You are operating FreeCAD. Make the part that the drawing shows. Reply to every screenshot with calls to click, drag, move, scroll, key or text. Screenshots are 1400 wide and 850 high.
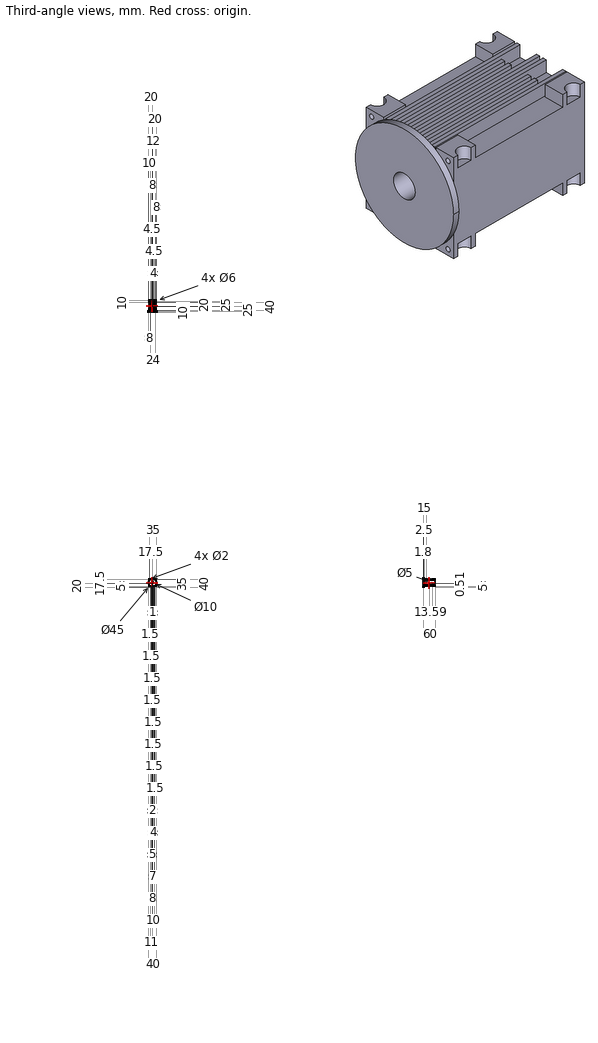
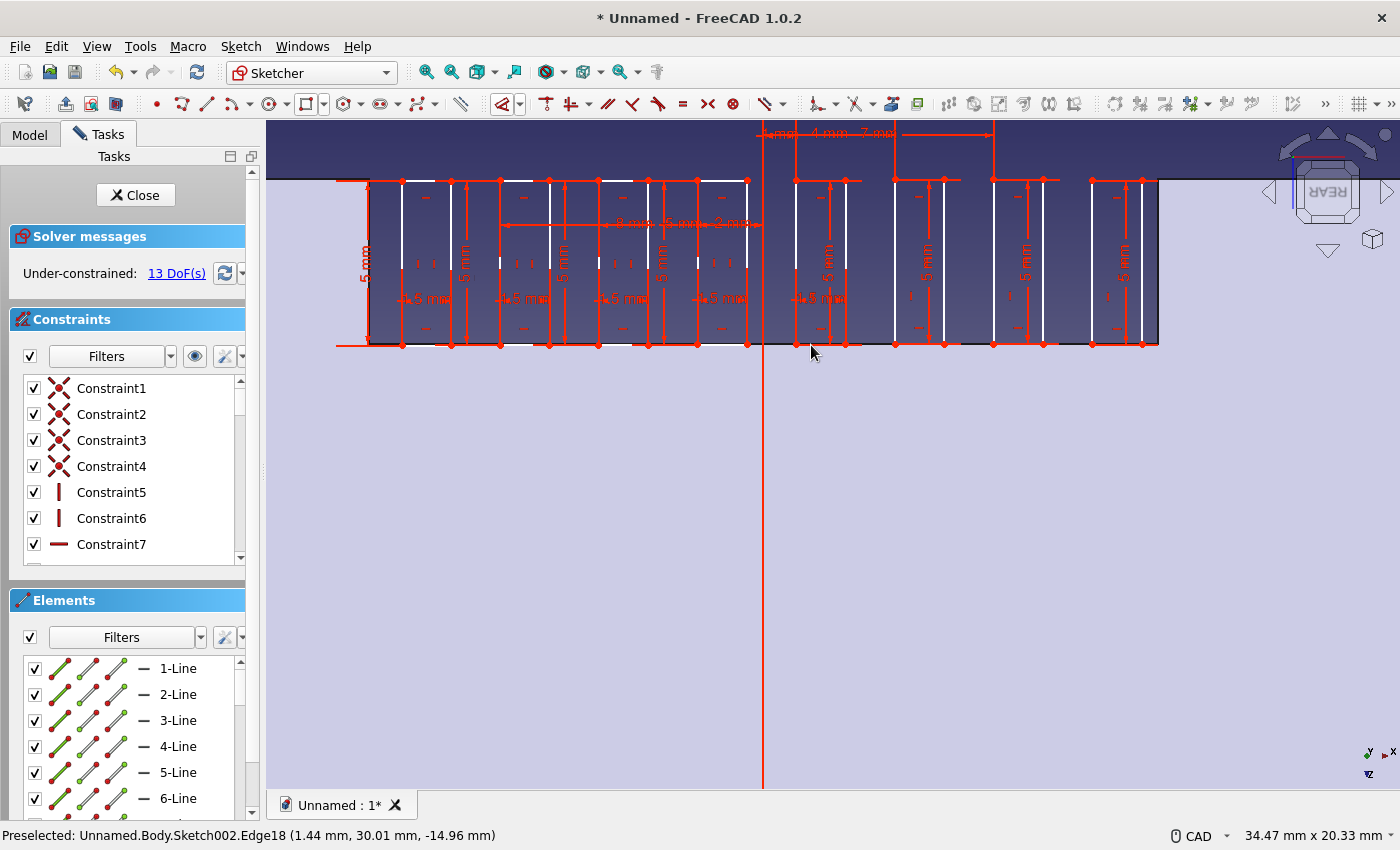
click(910, 344)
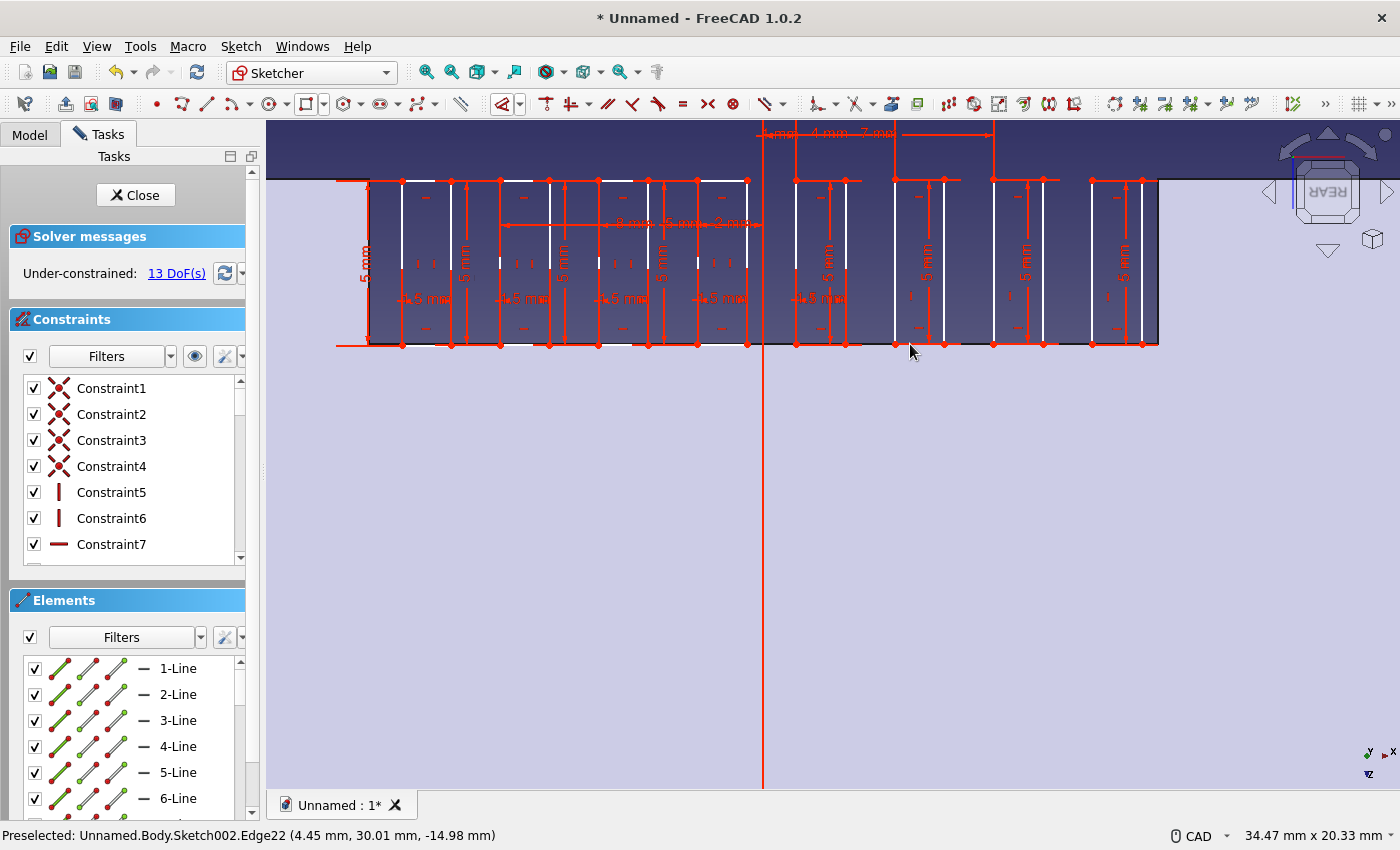
key(l)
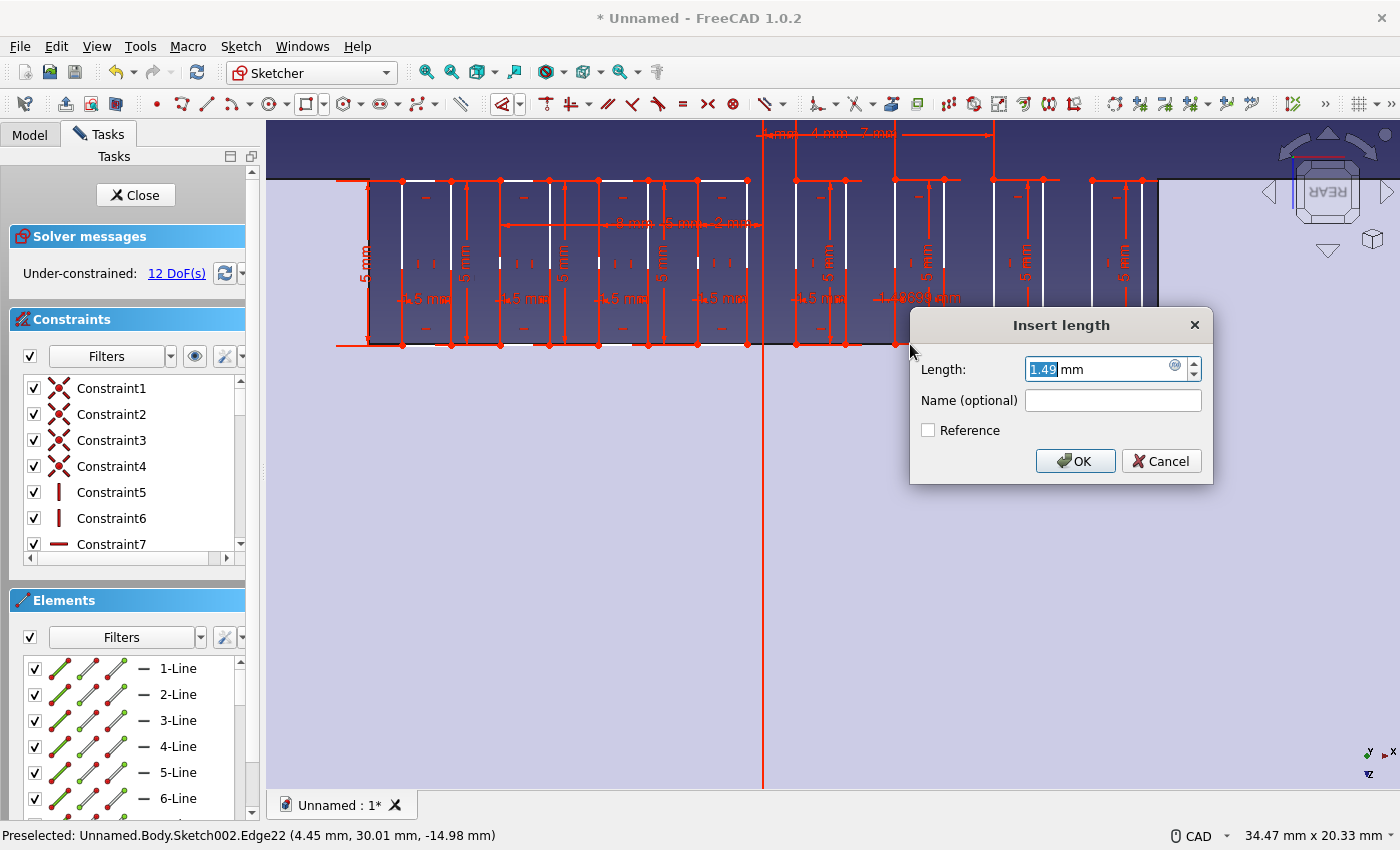
text(1.5)
key(Return)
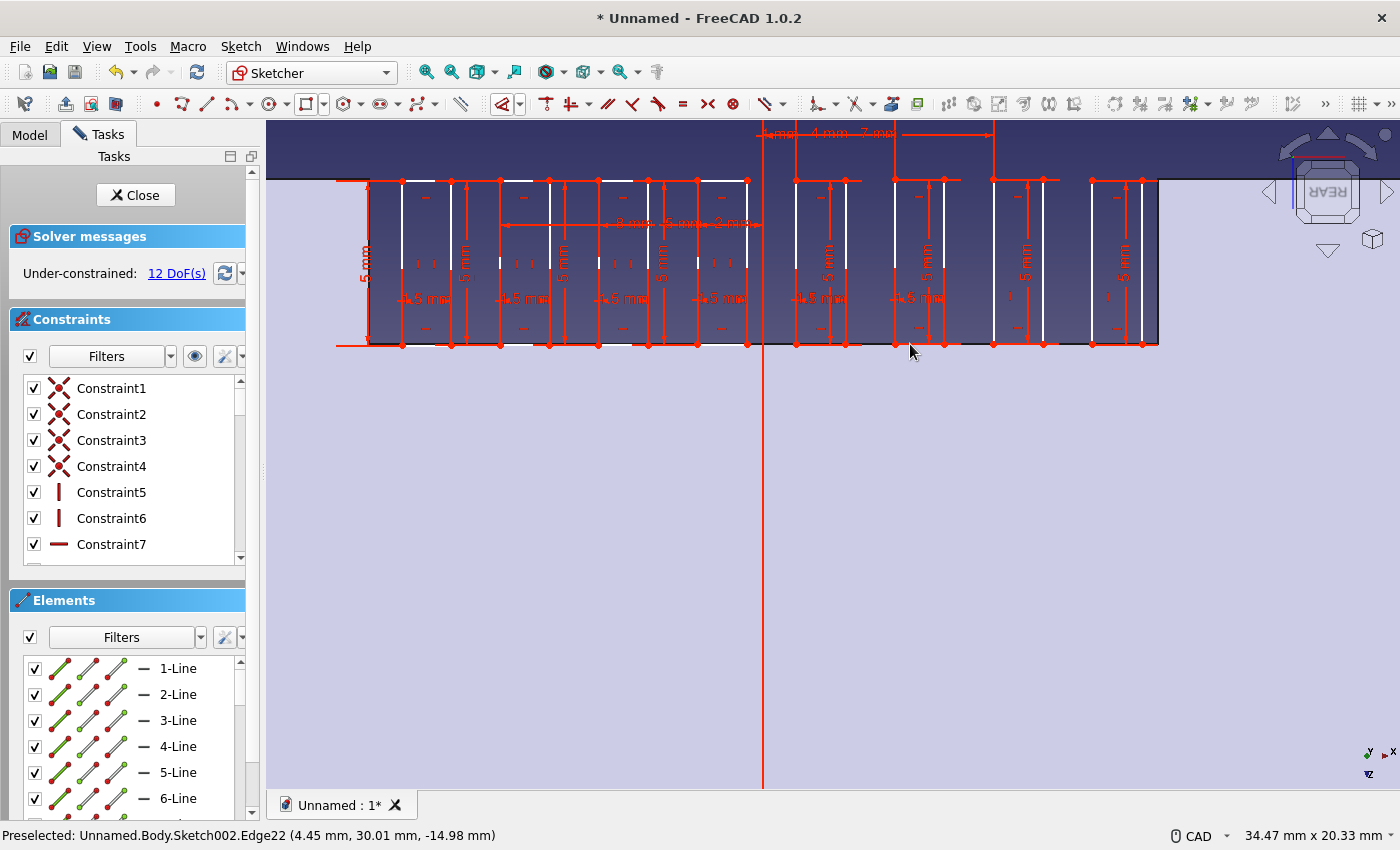
click(1009, 344)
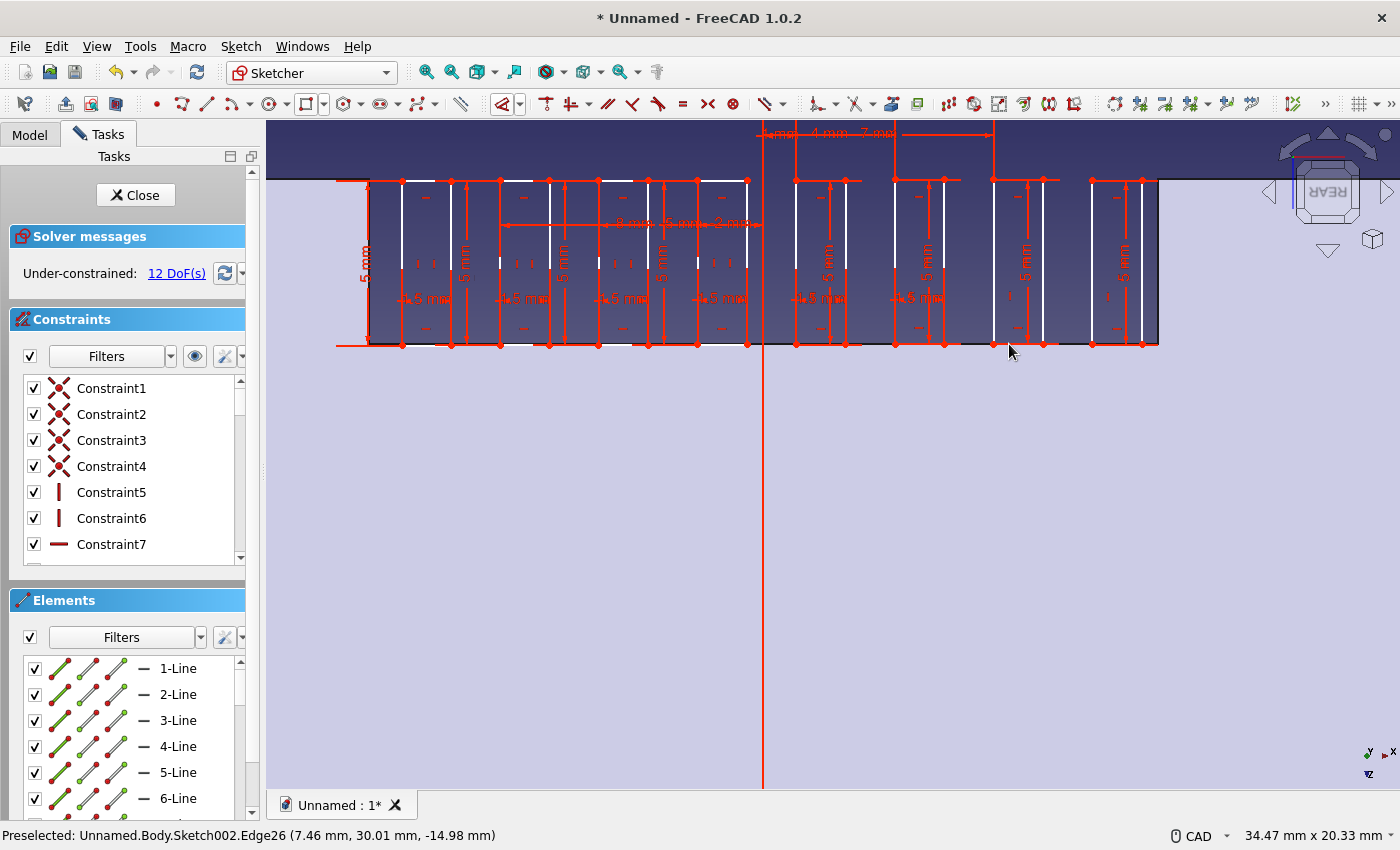
click(520, 104)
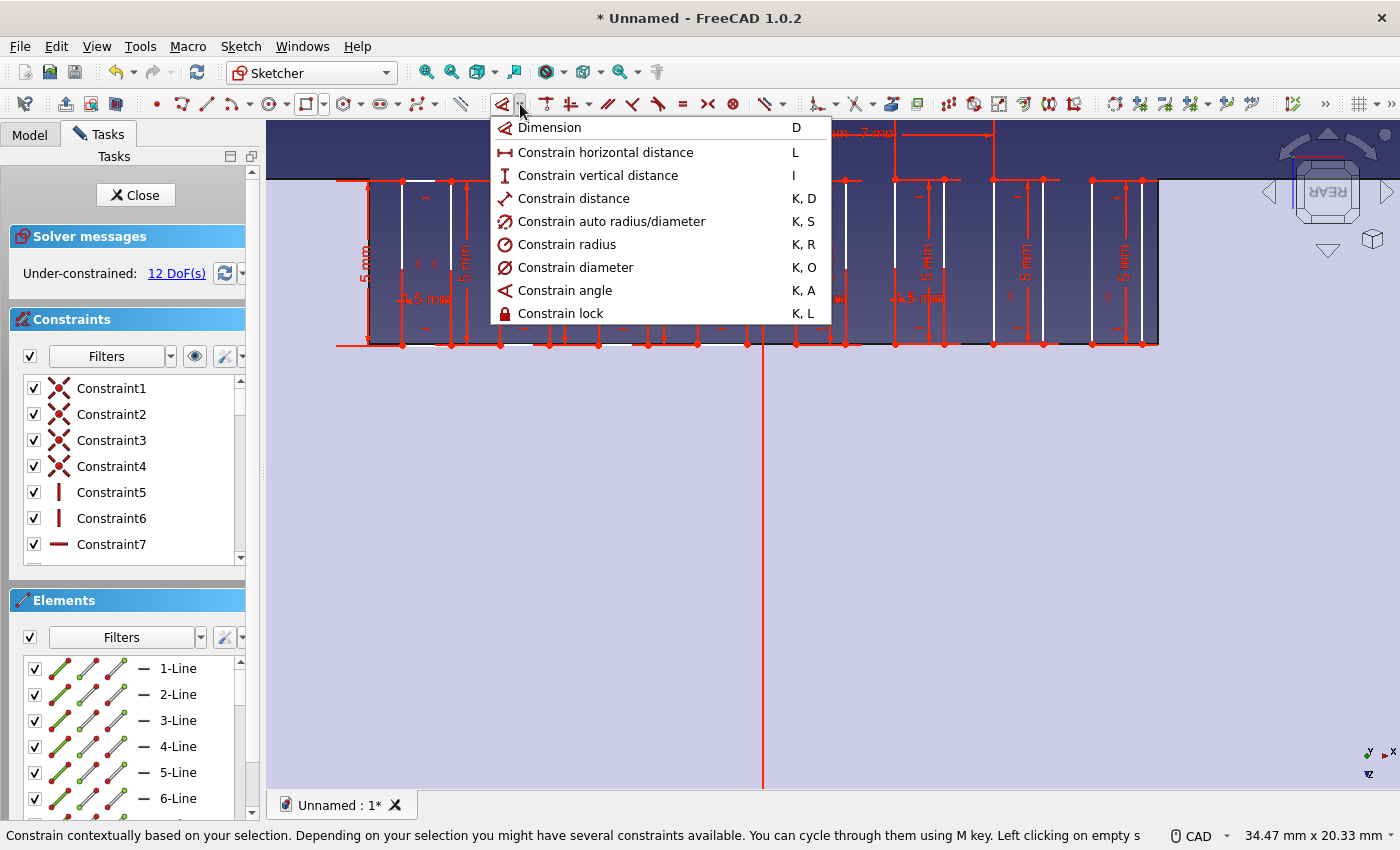
click(661, 152)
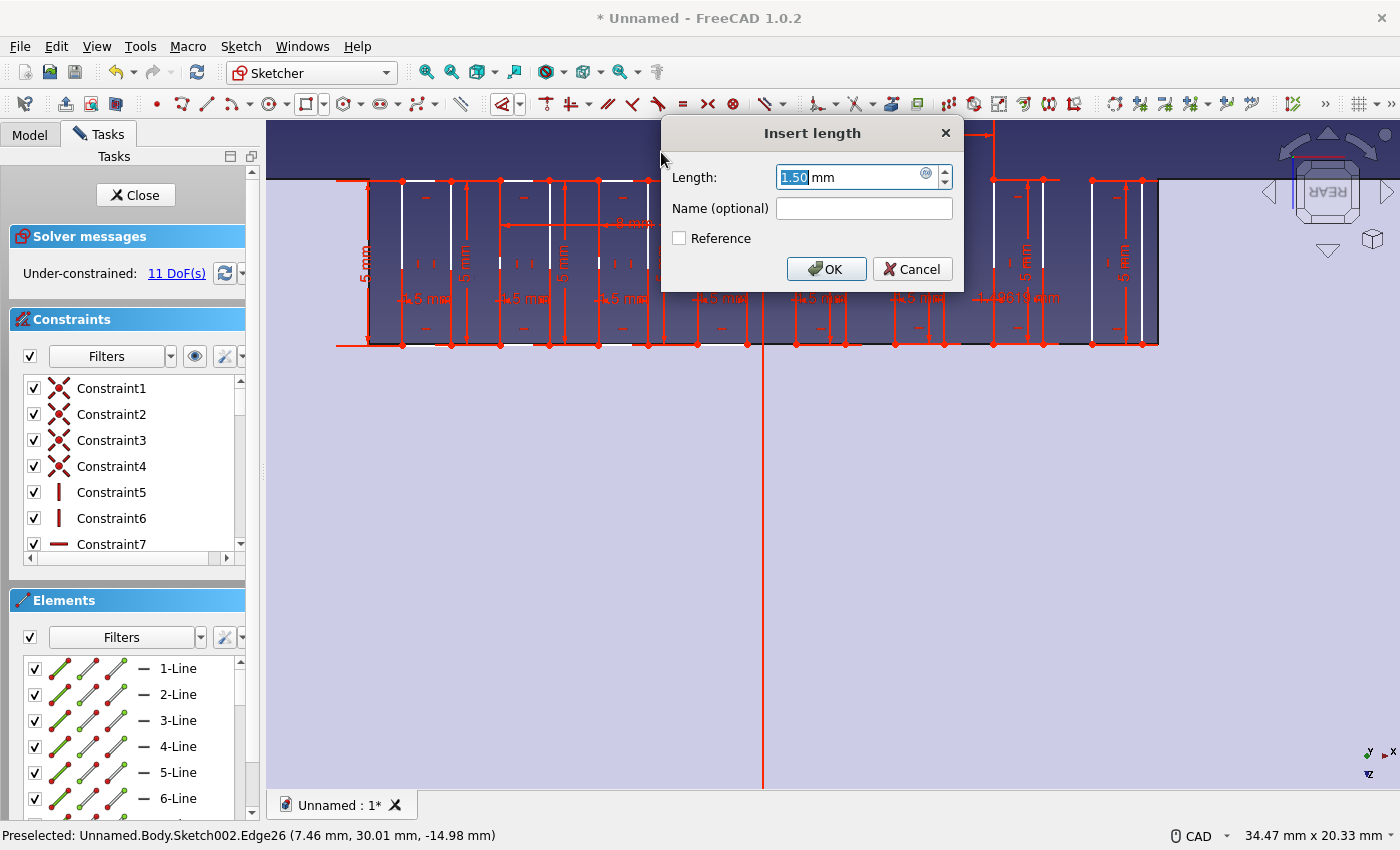
text(1.5)
key(Return)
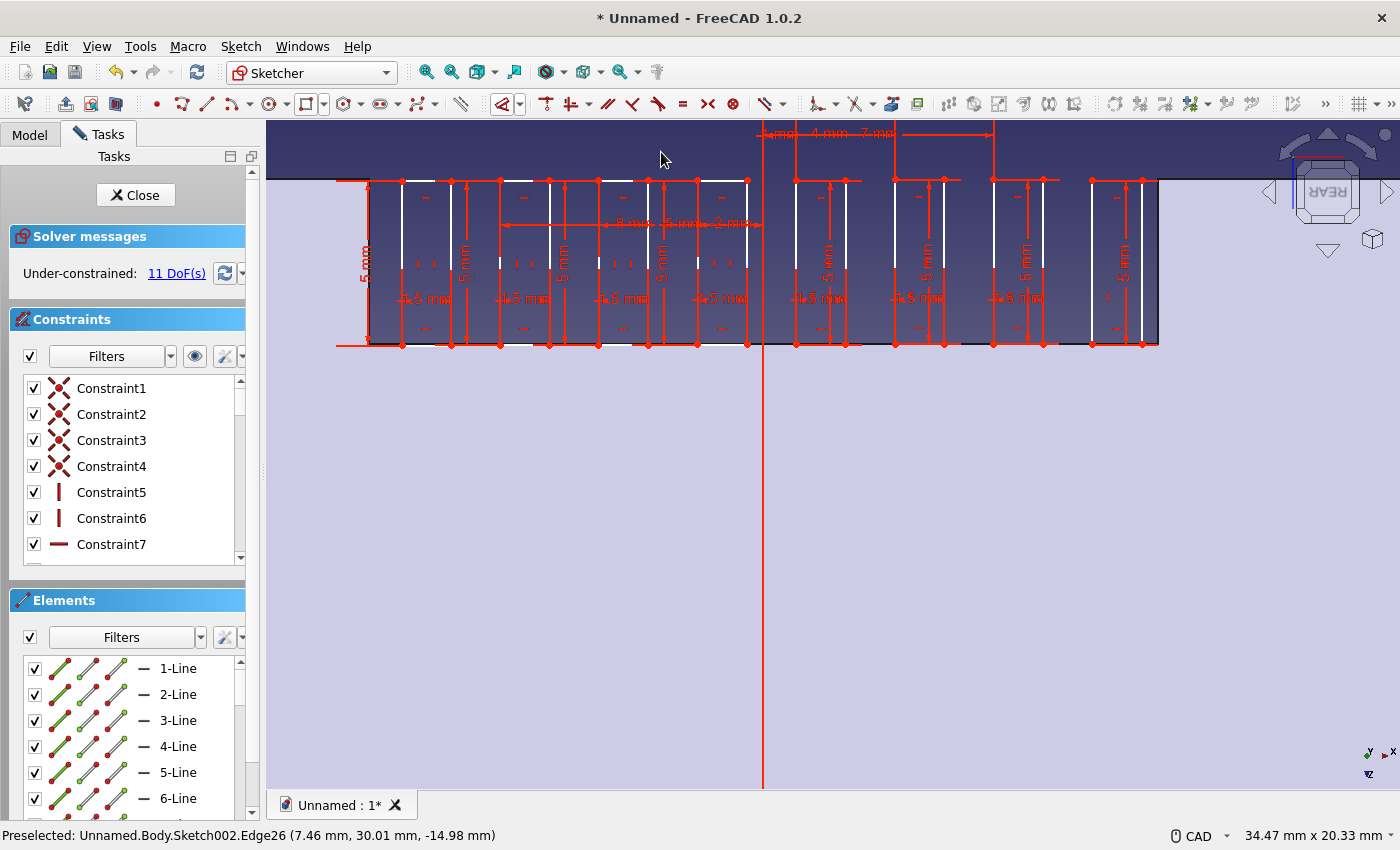
click(1107, 345)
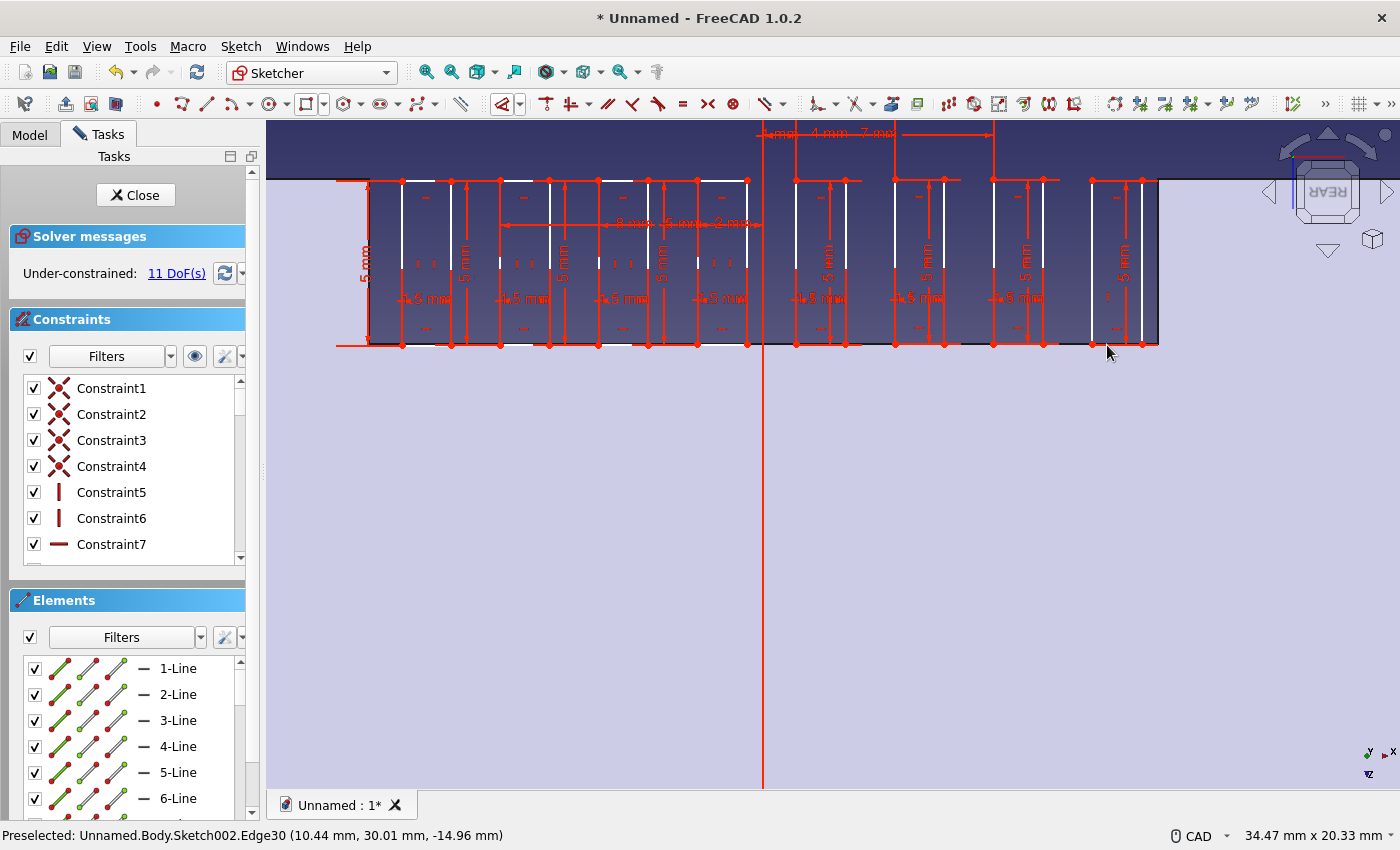
key(l)